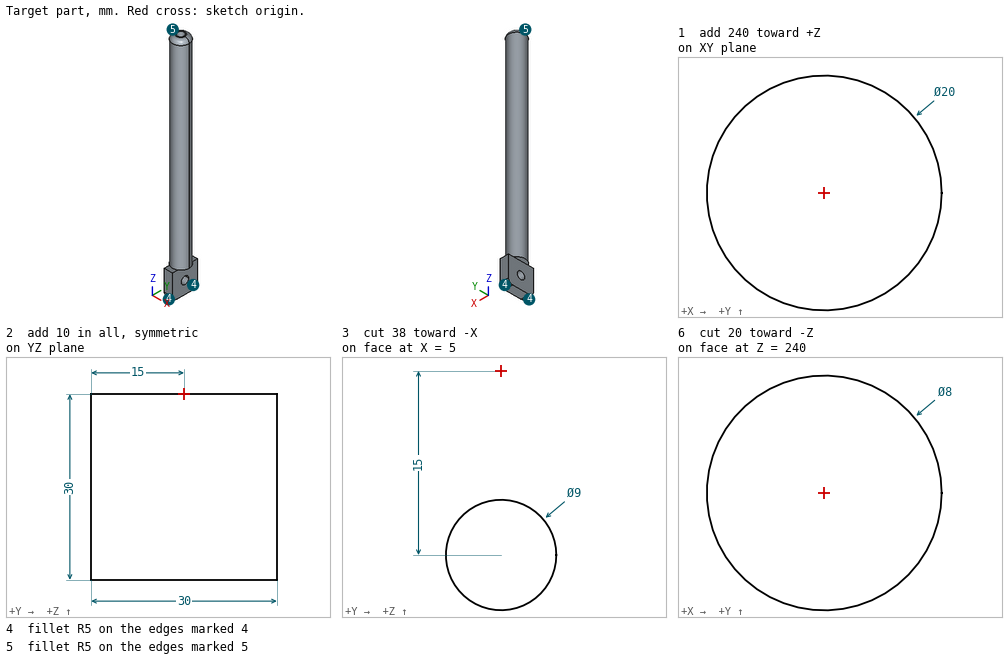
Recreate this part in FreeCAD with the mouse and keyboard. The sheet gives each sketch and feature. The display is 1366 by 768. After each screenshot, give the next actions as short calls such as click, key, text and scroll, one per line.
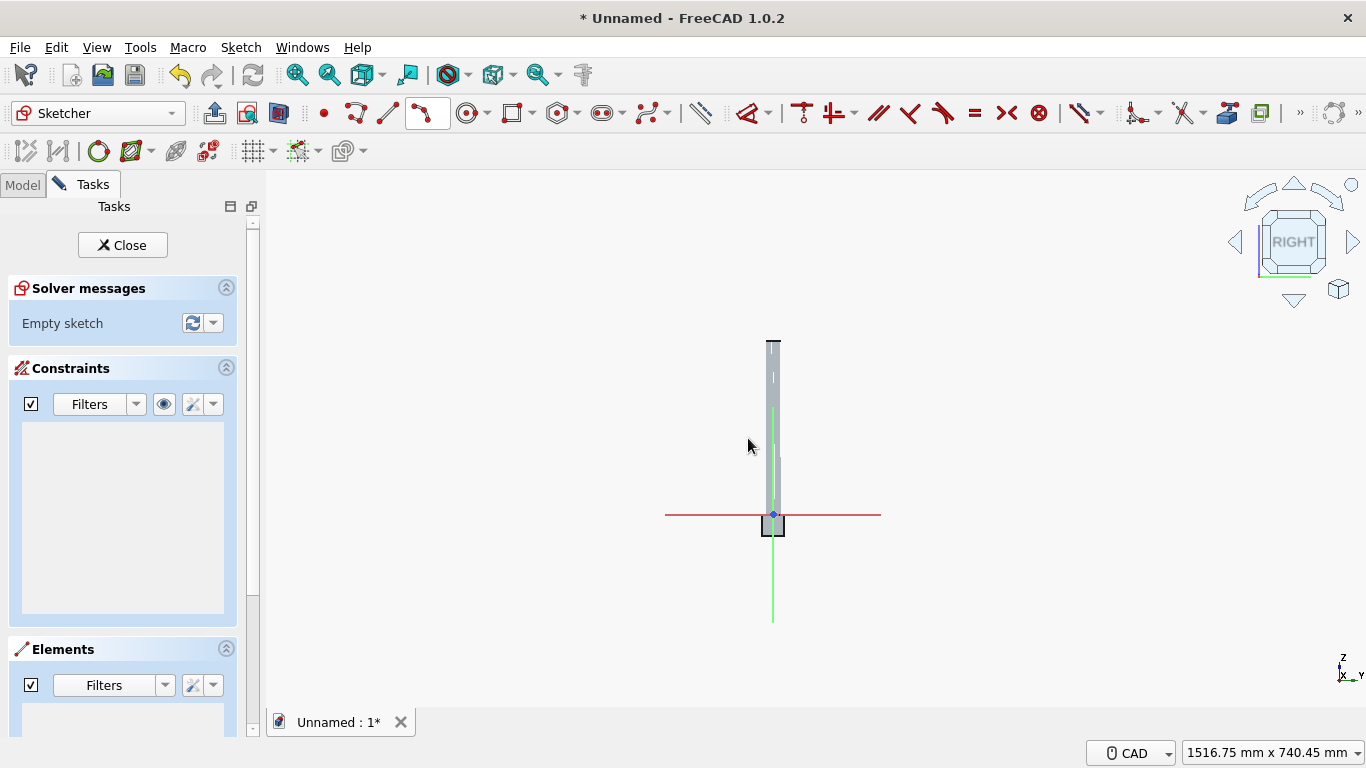
scroll(775, 526, up, 15)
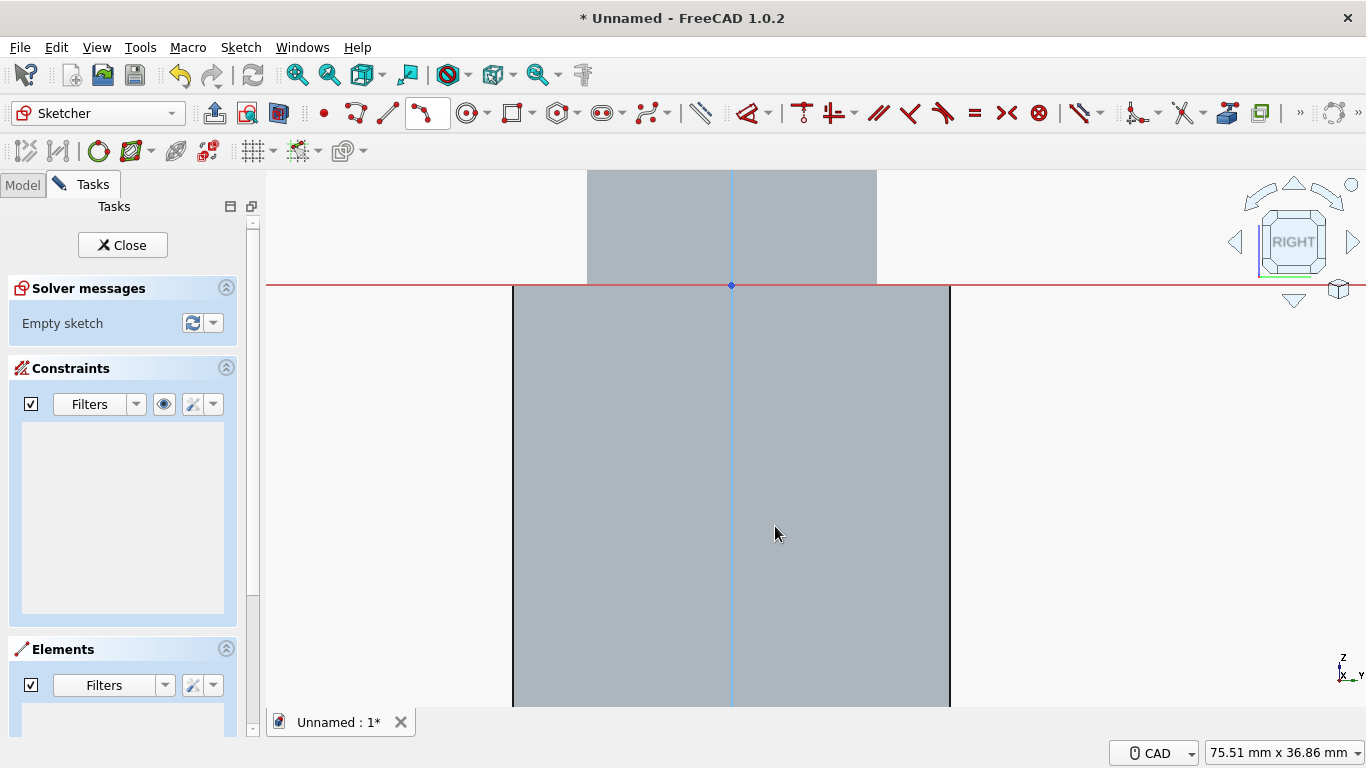
key(g)
key(c)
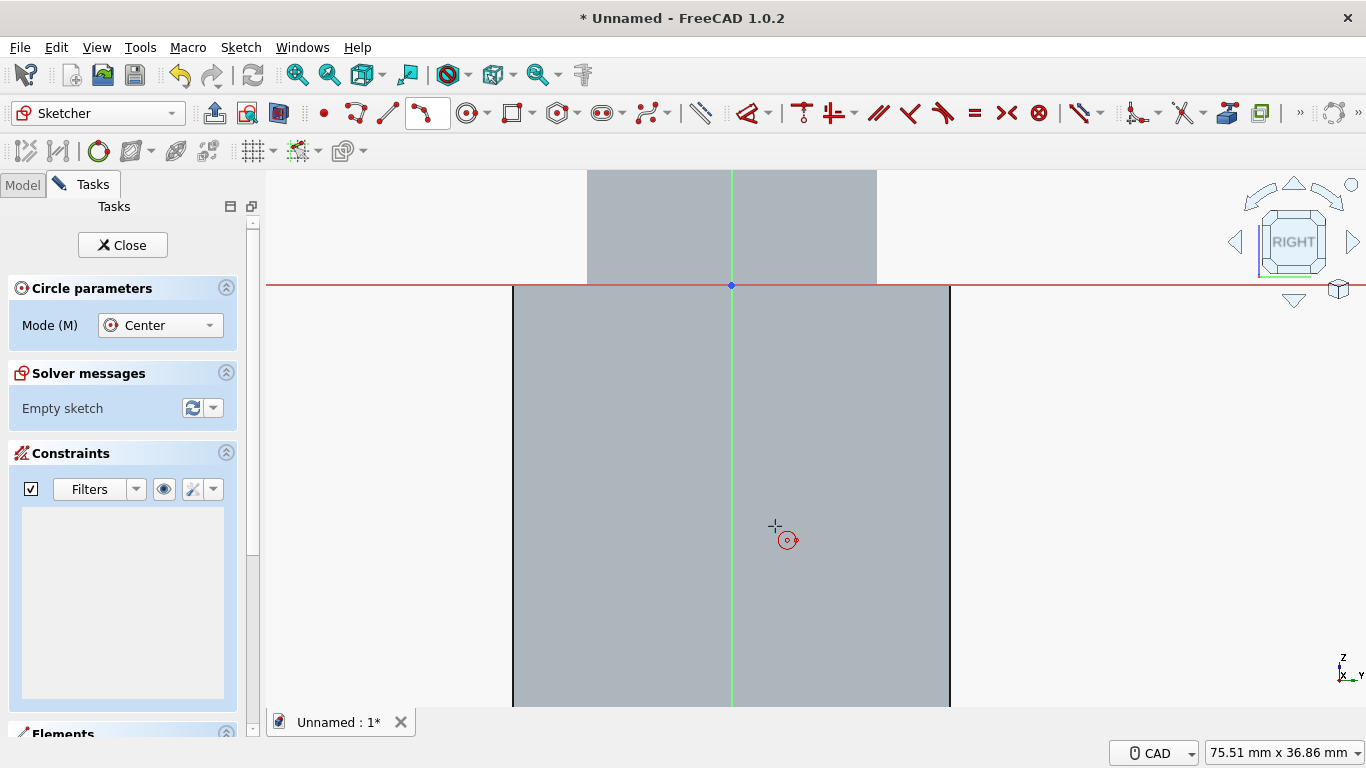
click(732, 504)
click(778, 457)
key(Escape)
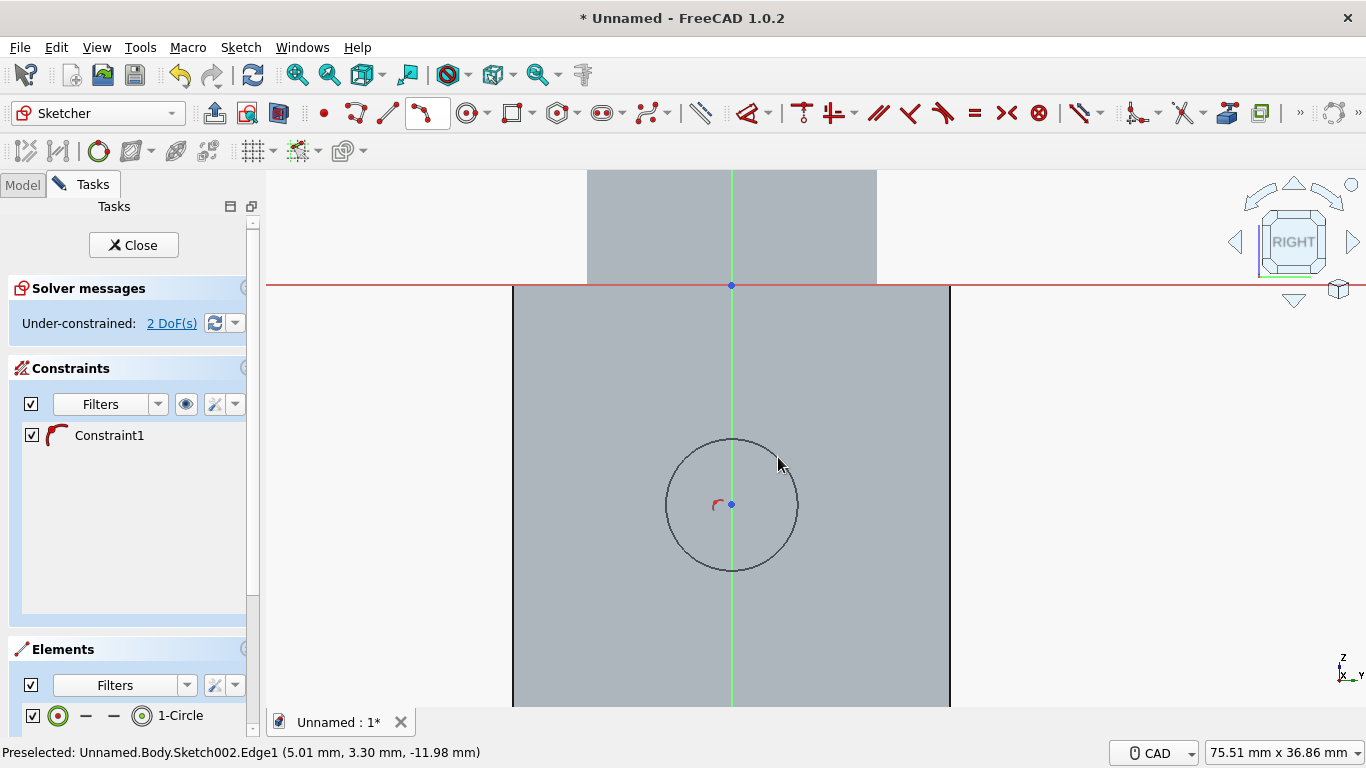
key(d)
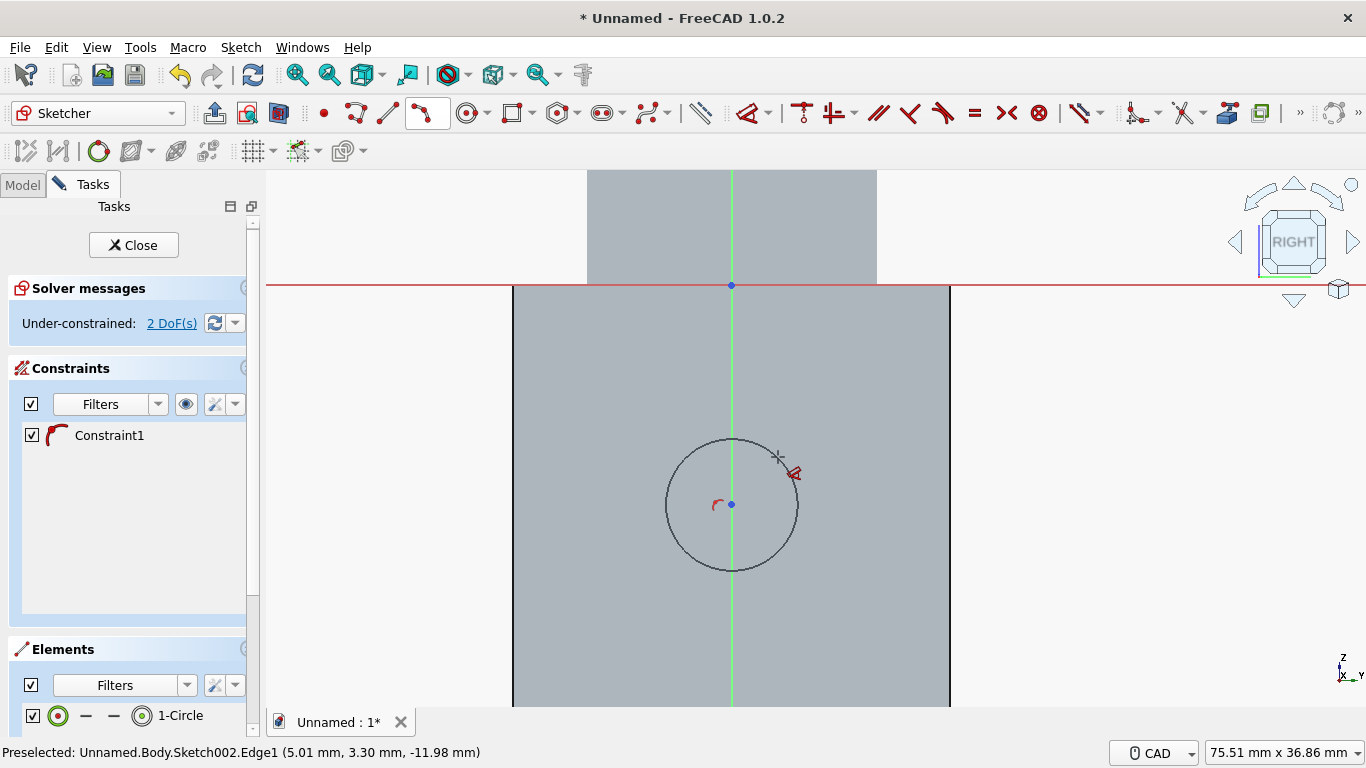
click(778, 458)
click(800, 435)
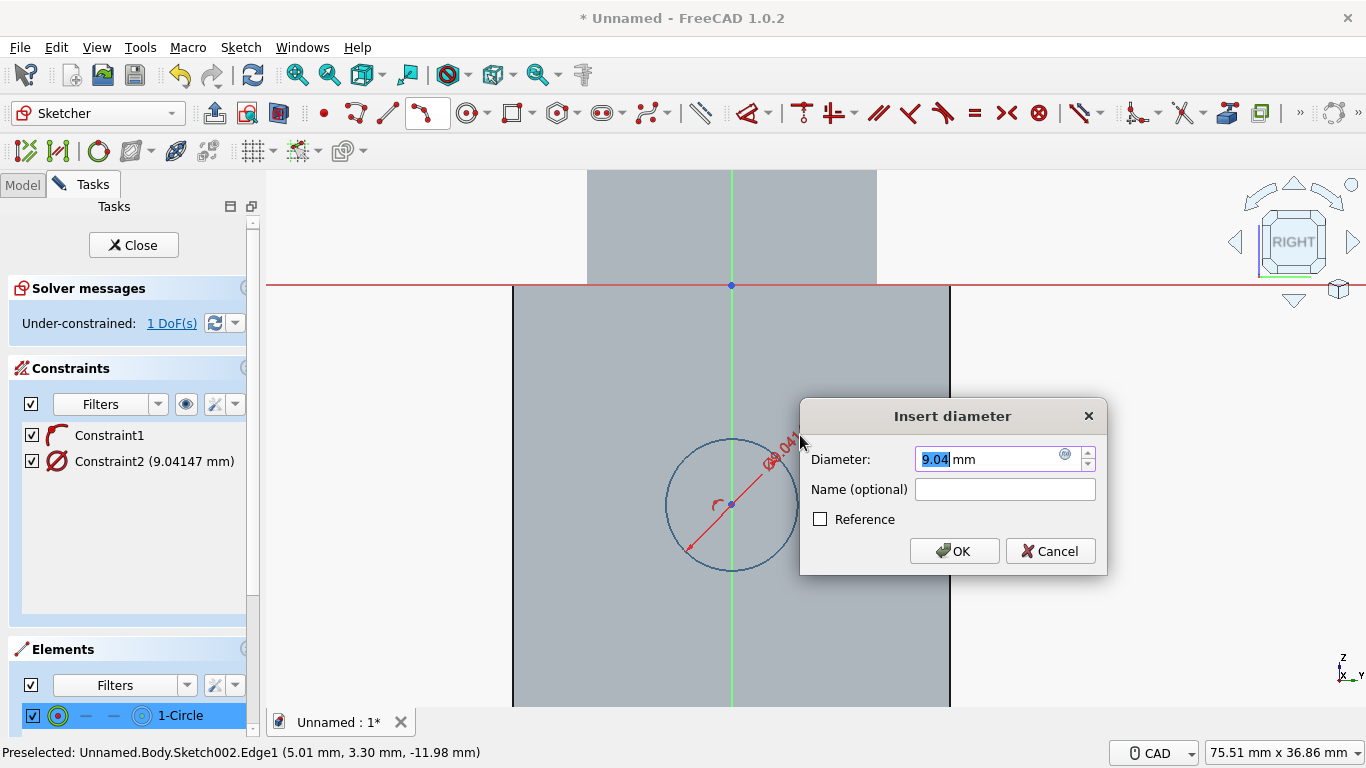
text(9)
key(Return)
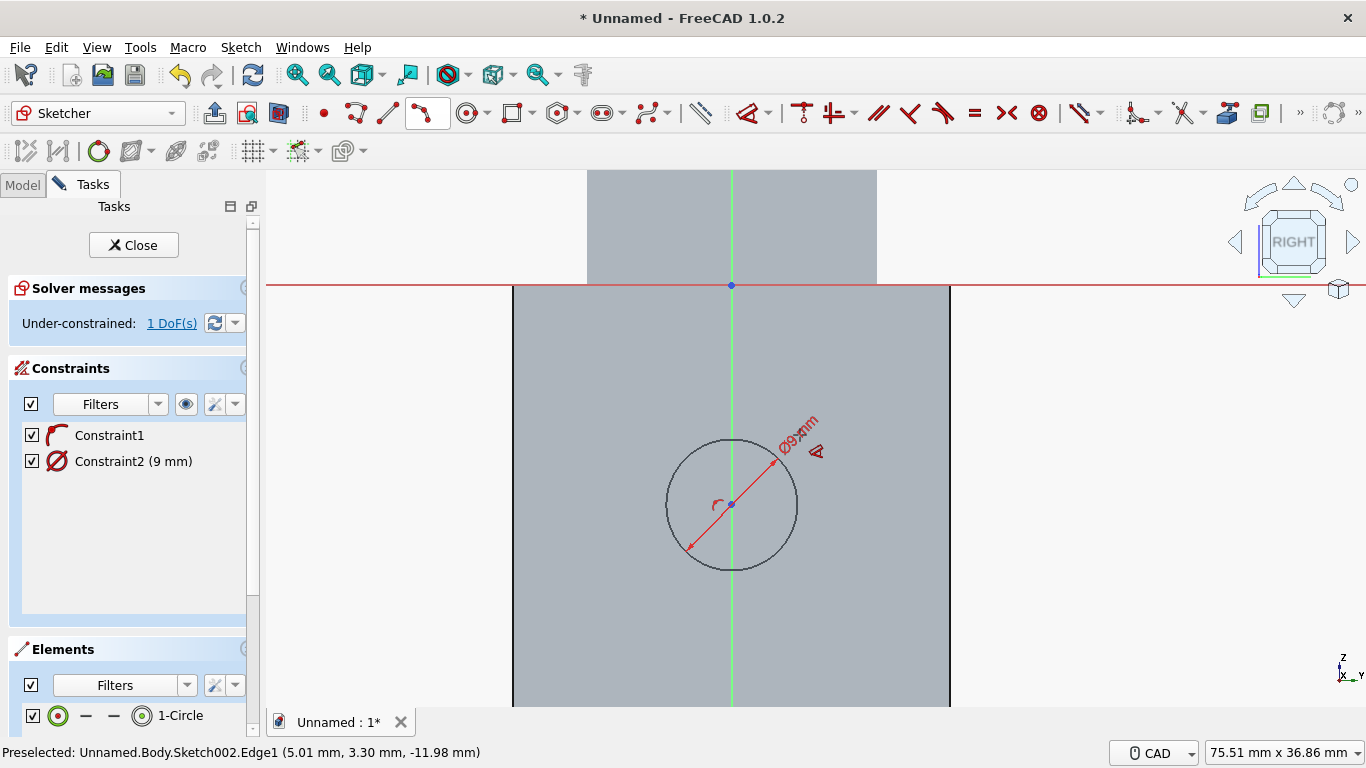
click(732, 505)
click(766, 395)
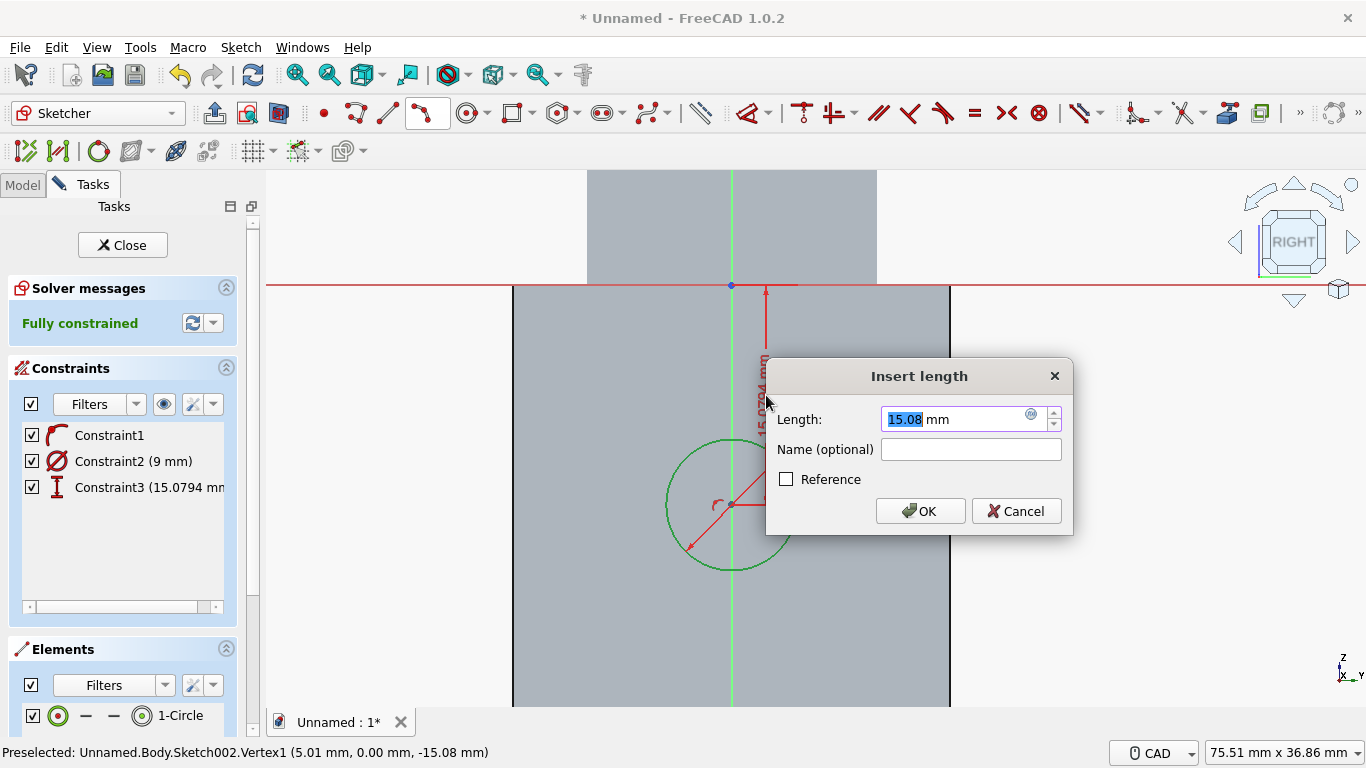
text(15)
key(Return)
key(Escape)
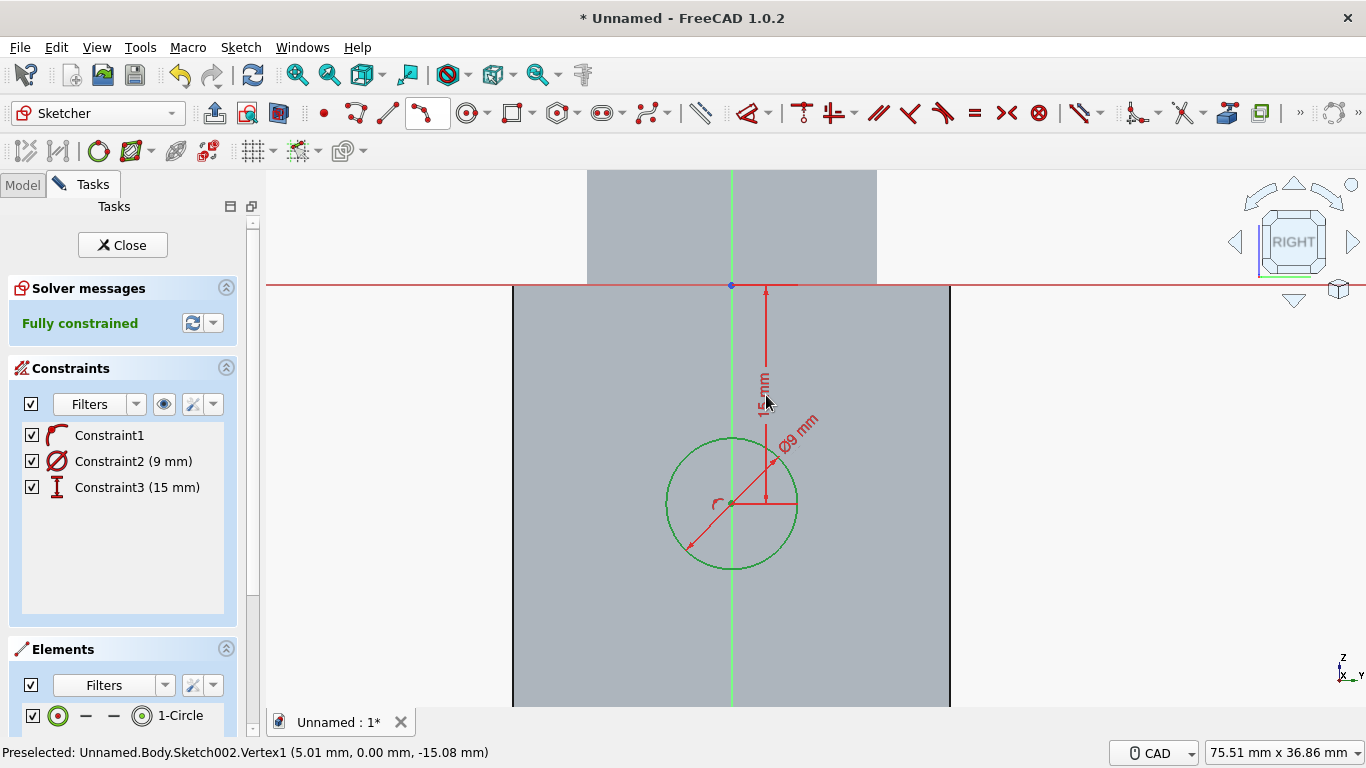
click(123, 245)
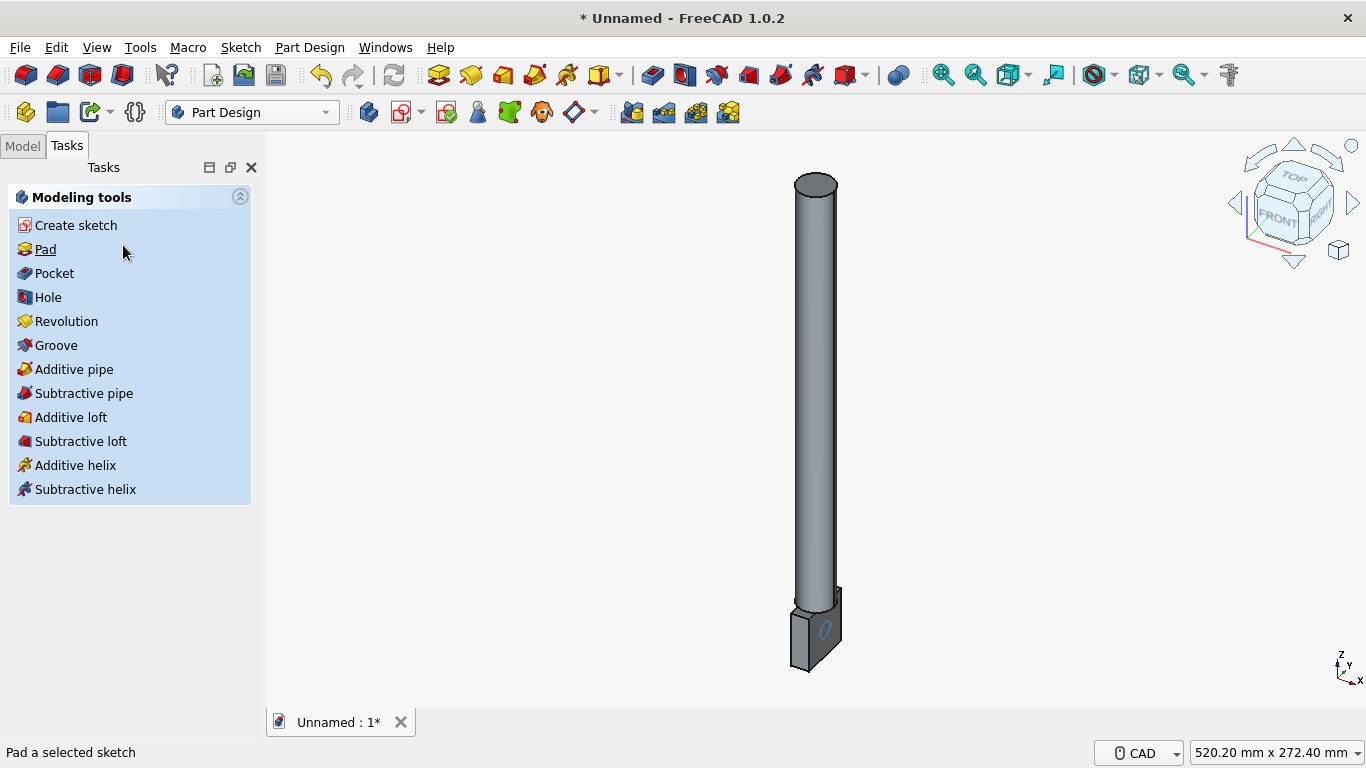
click(654, 76)